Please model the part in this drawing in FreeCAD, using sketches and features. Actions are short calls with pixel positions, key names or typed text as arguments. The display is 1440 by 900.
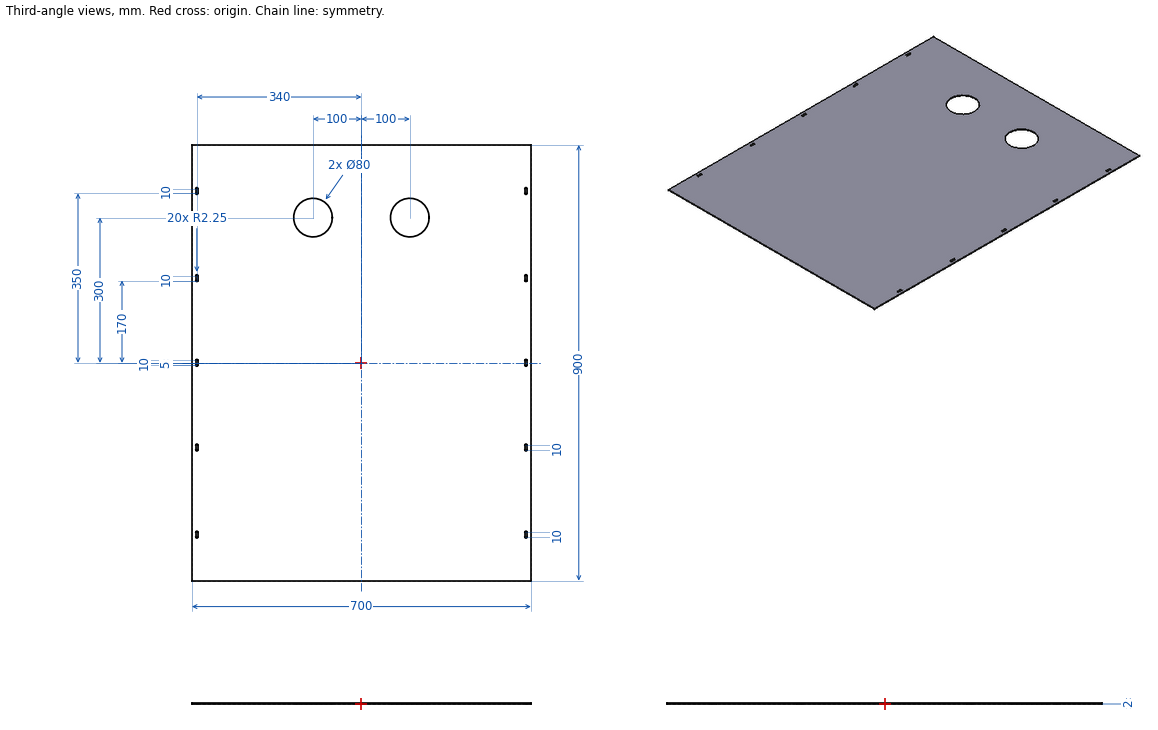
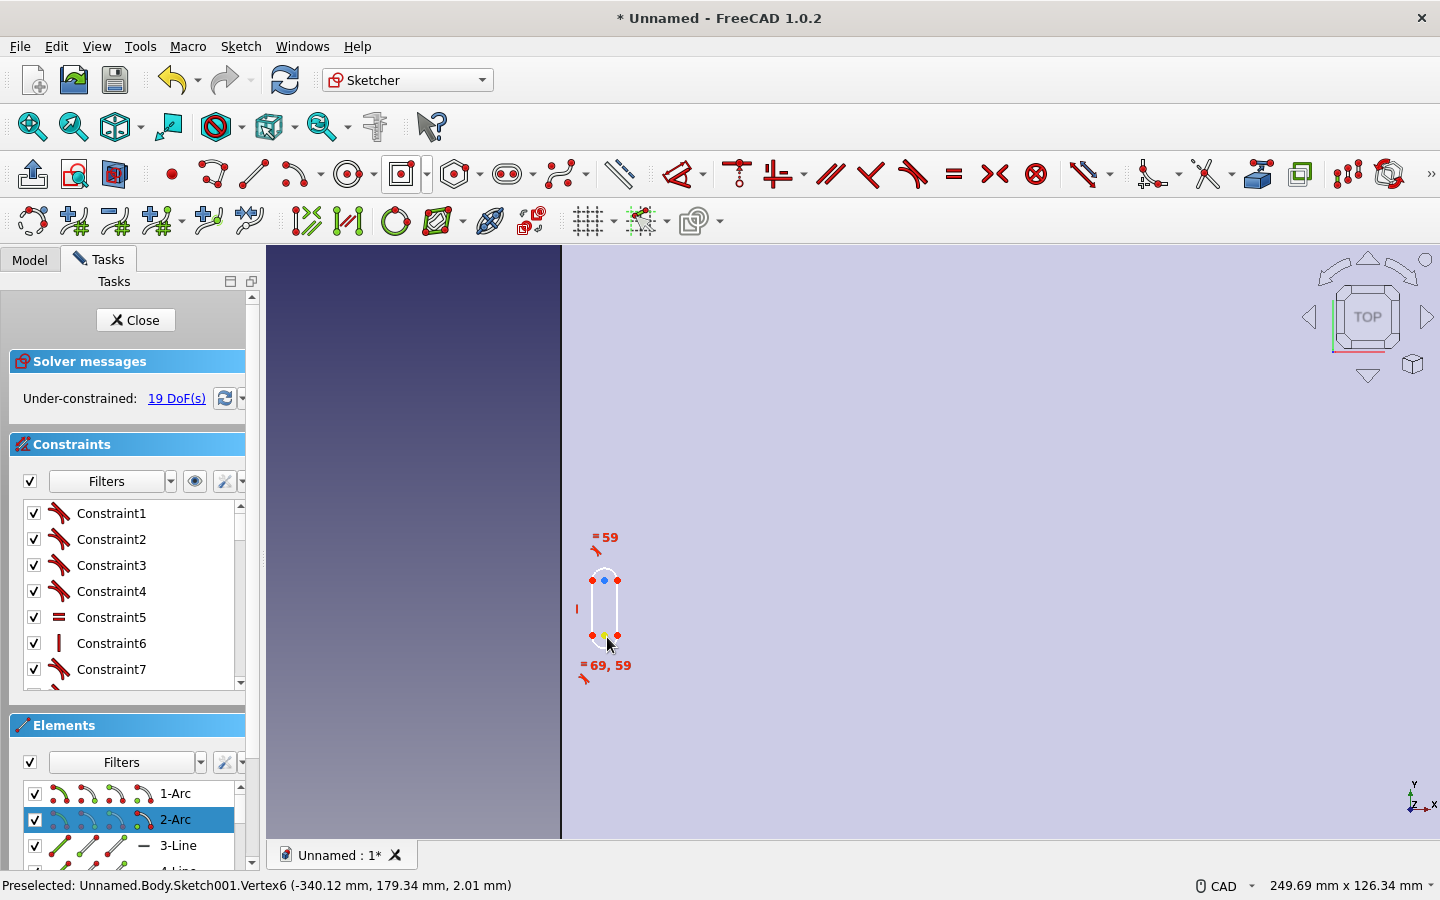
click(605, 636)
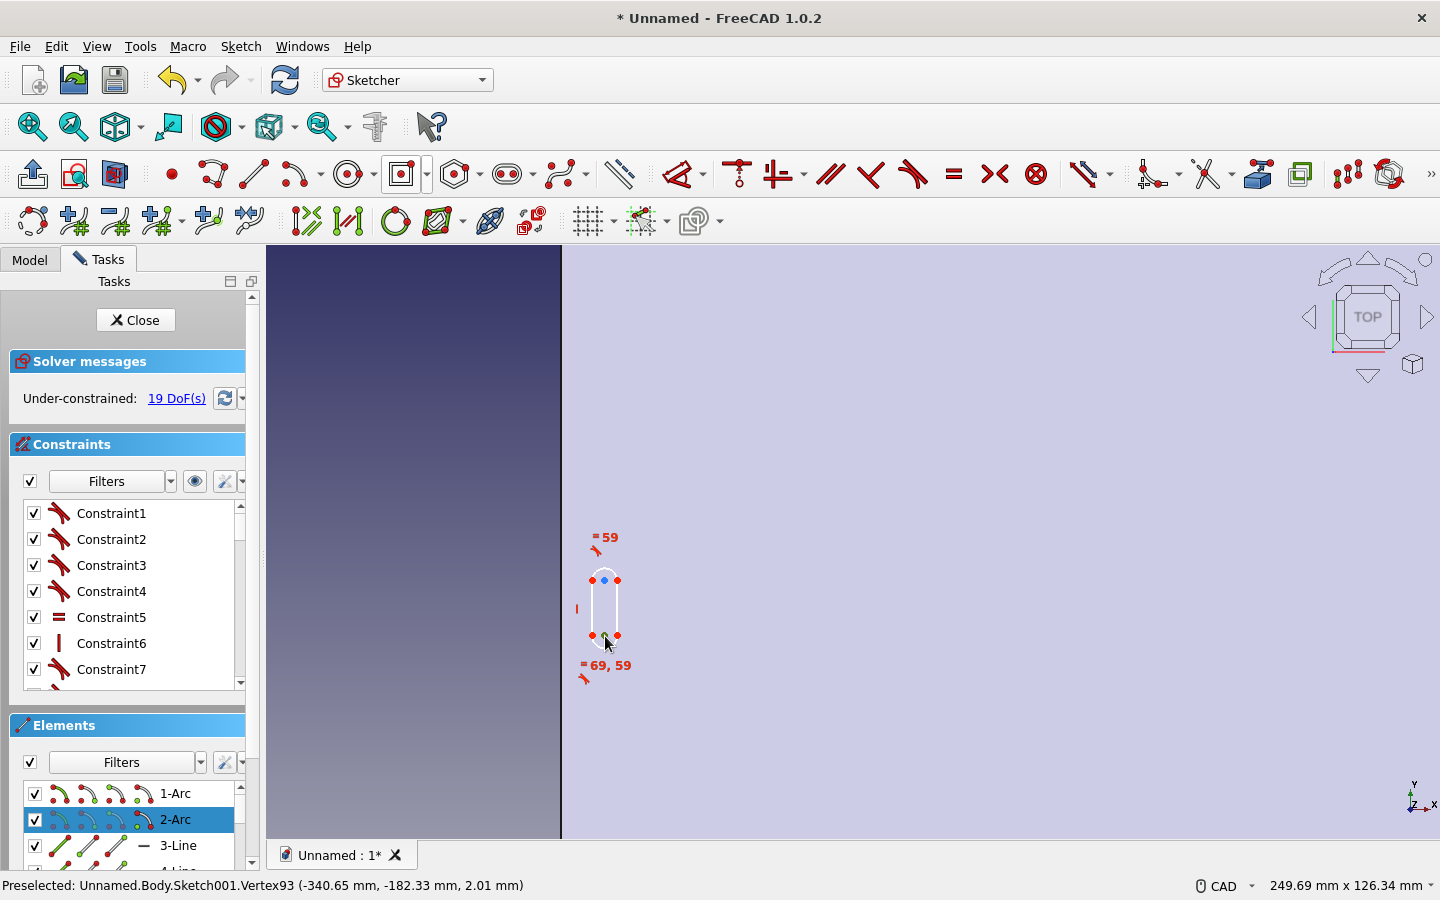
scroll(607, 637, down, 11)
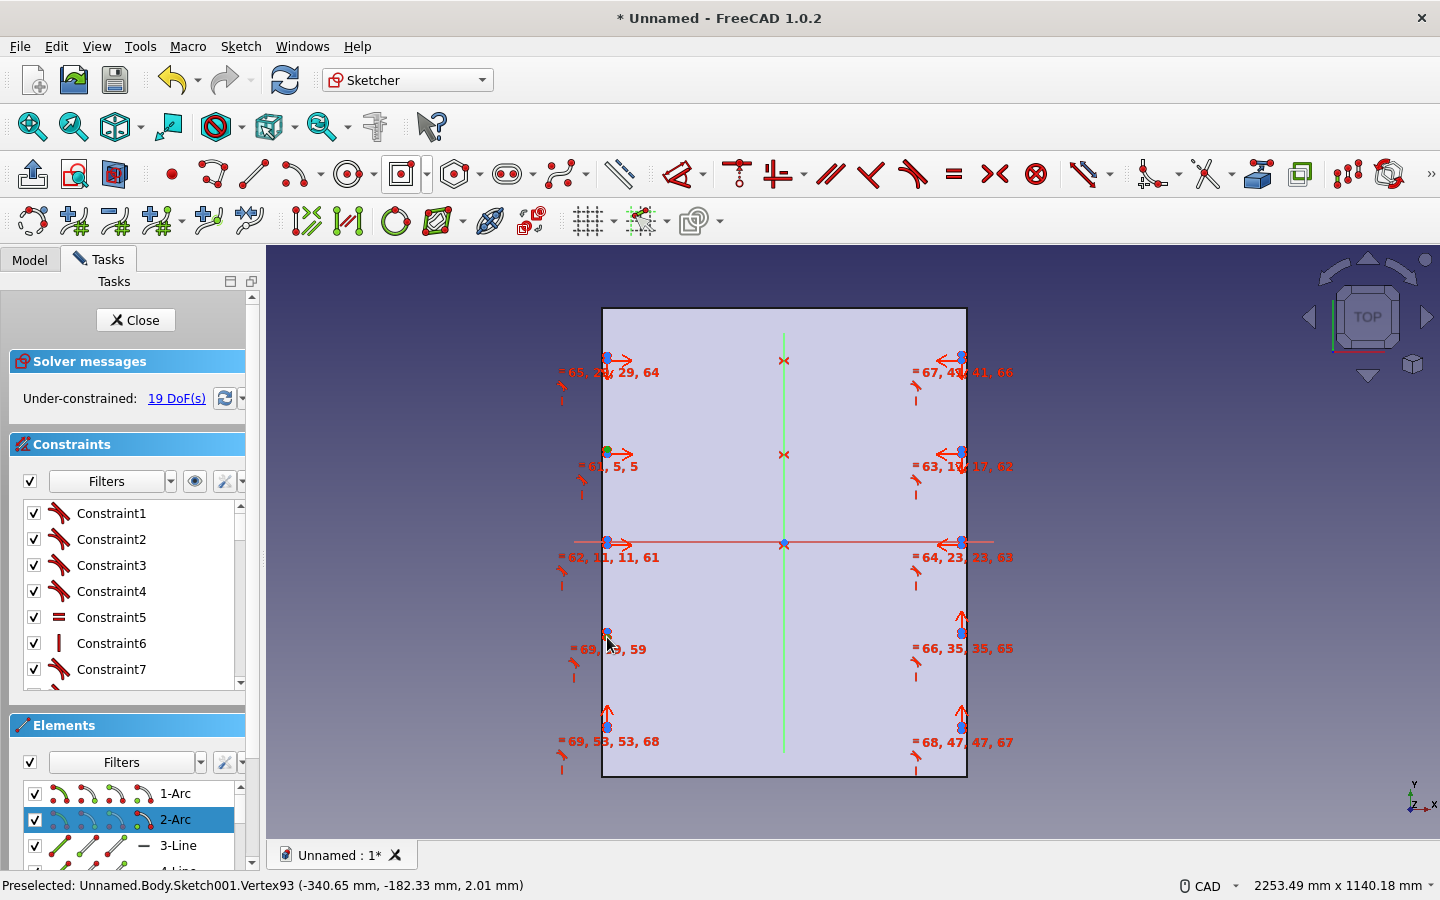
click(574, 542)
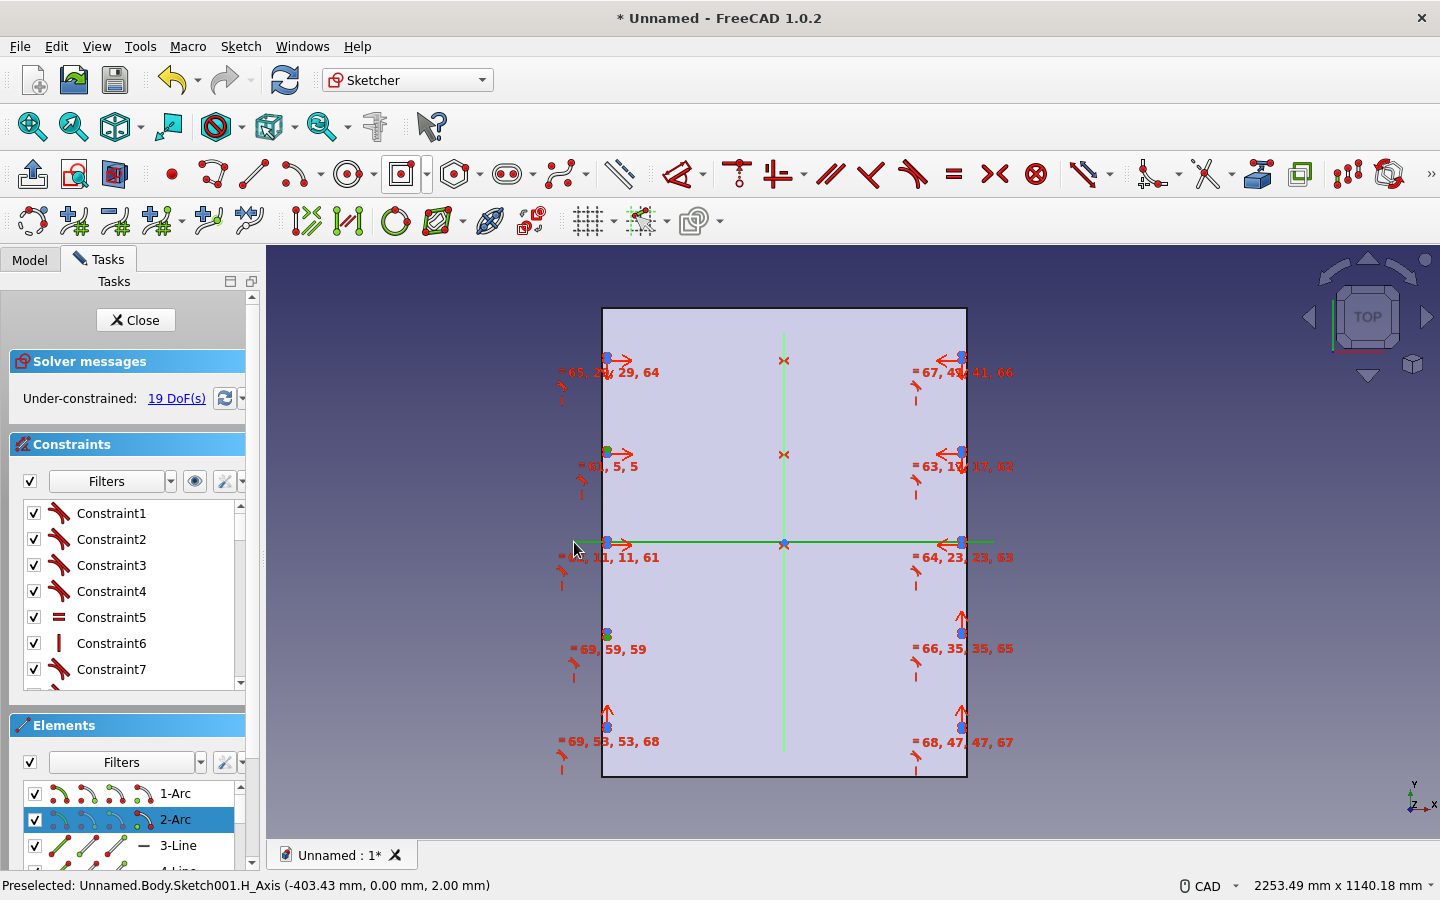
key(s)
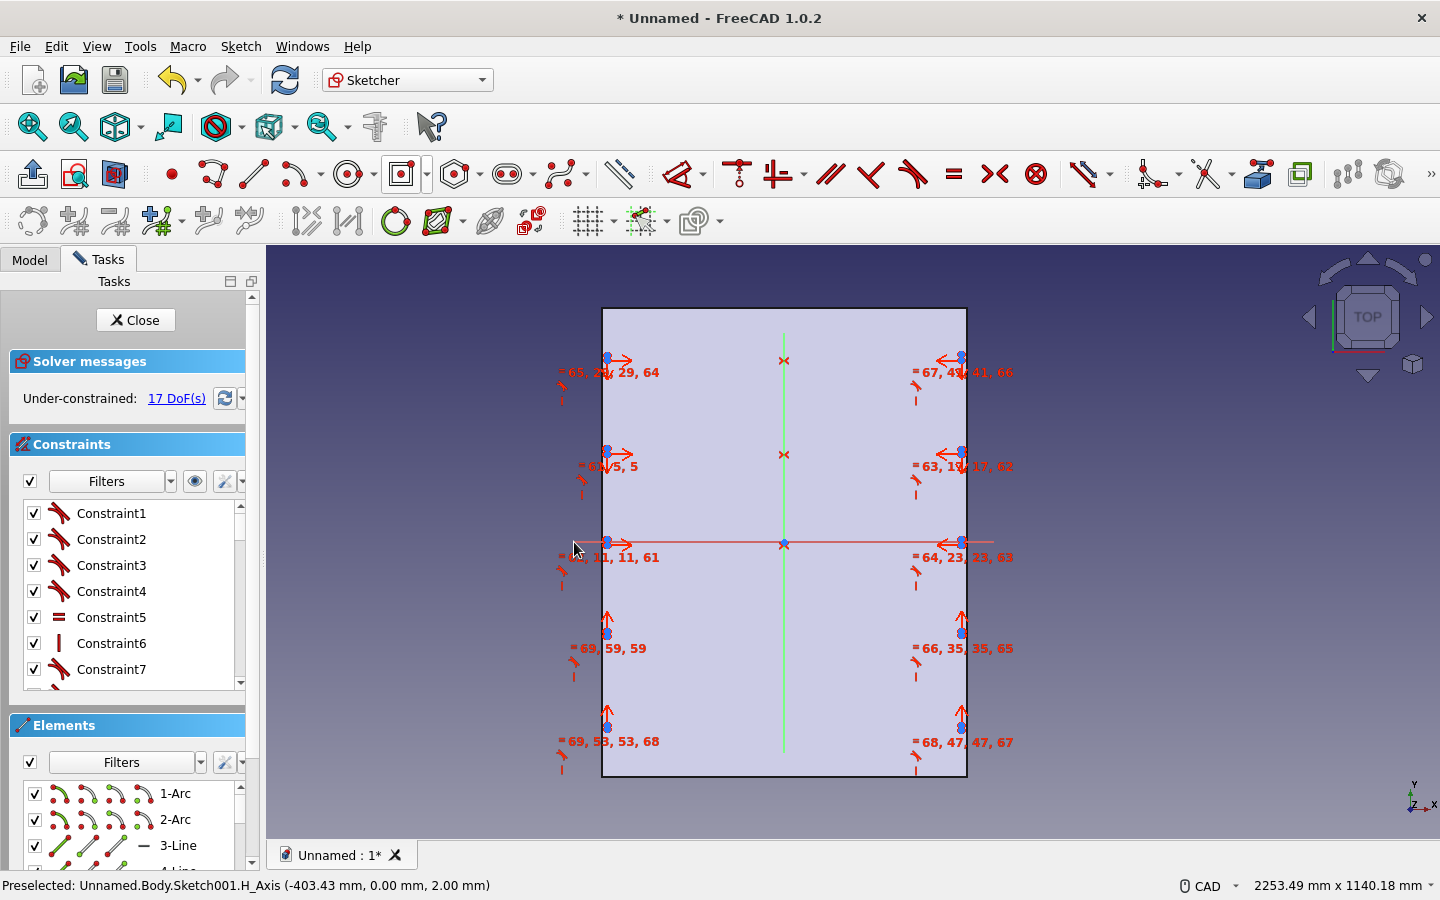
key(d)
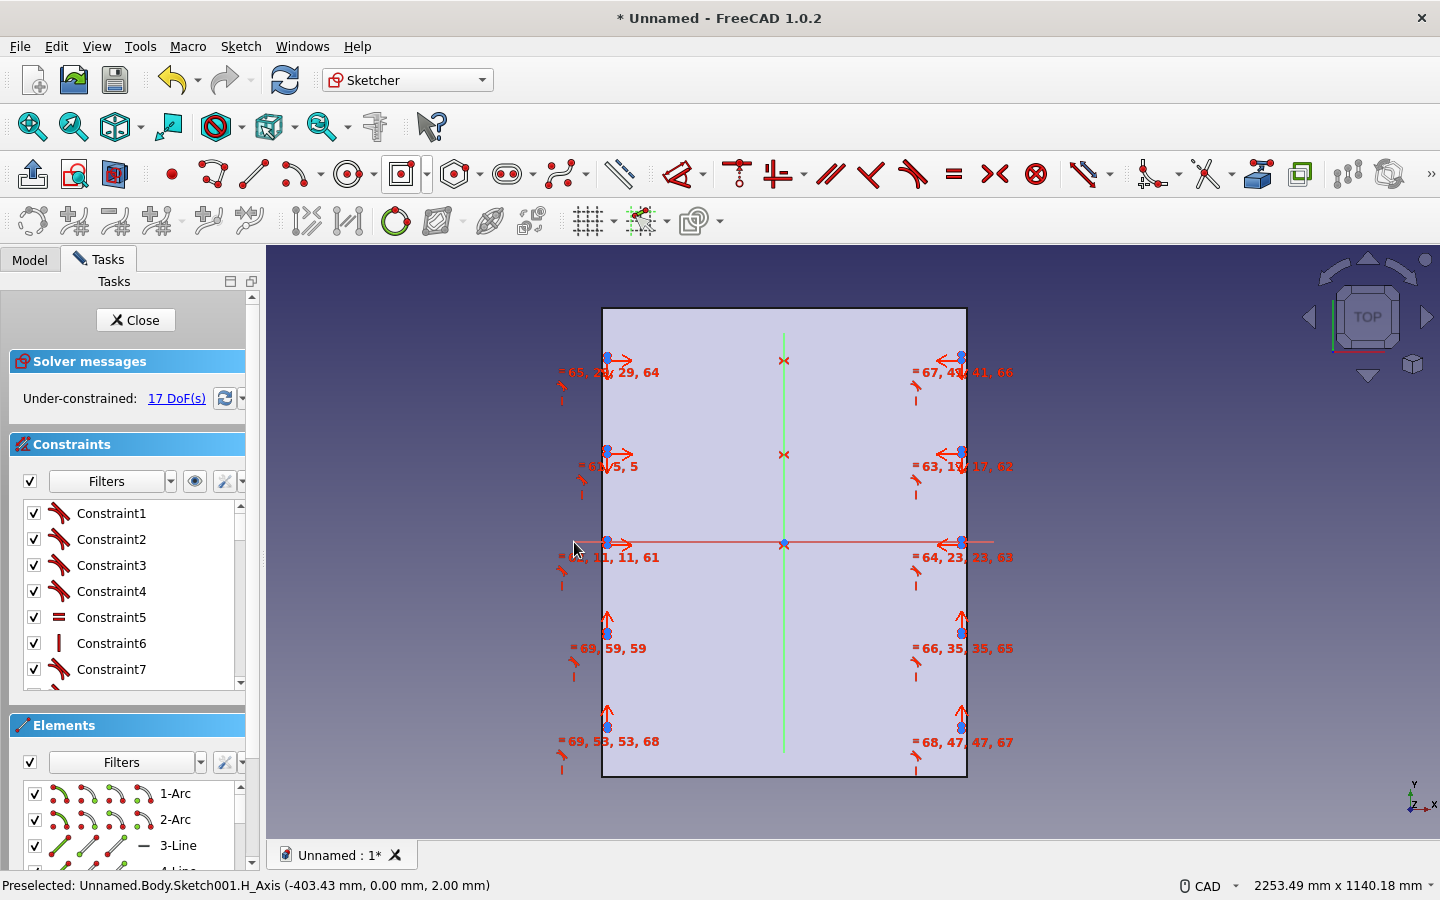
scroll(607, 456, up, 18)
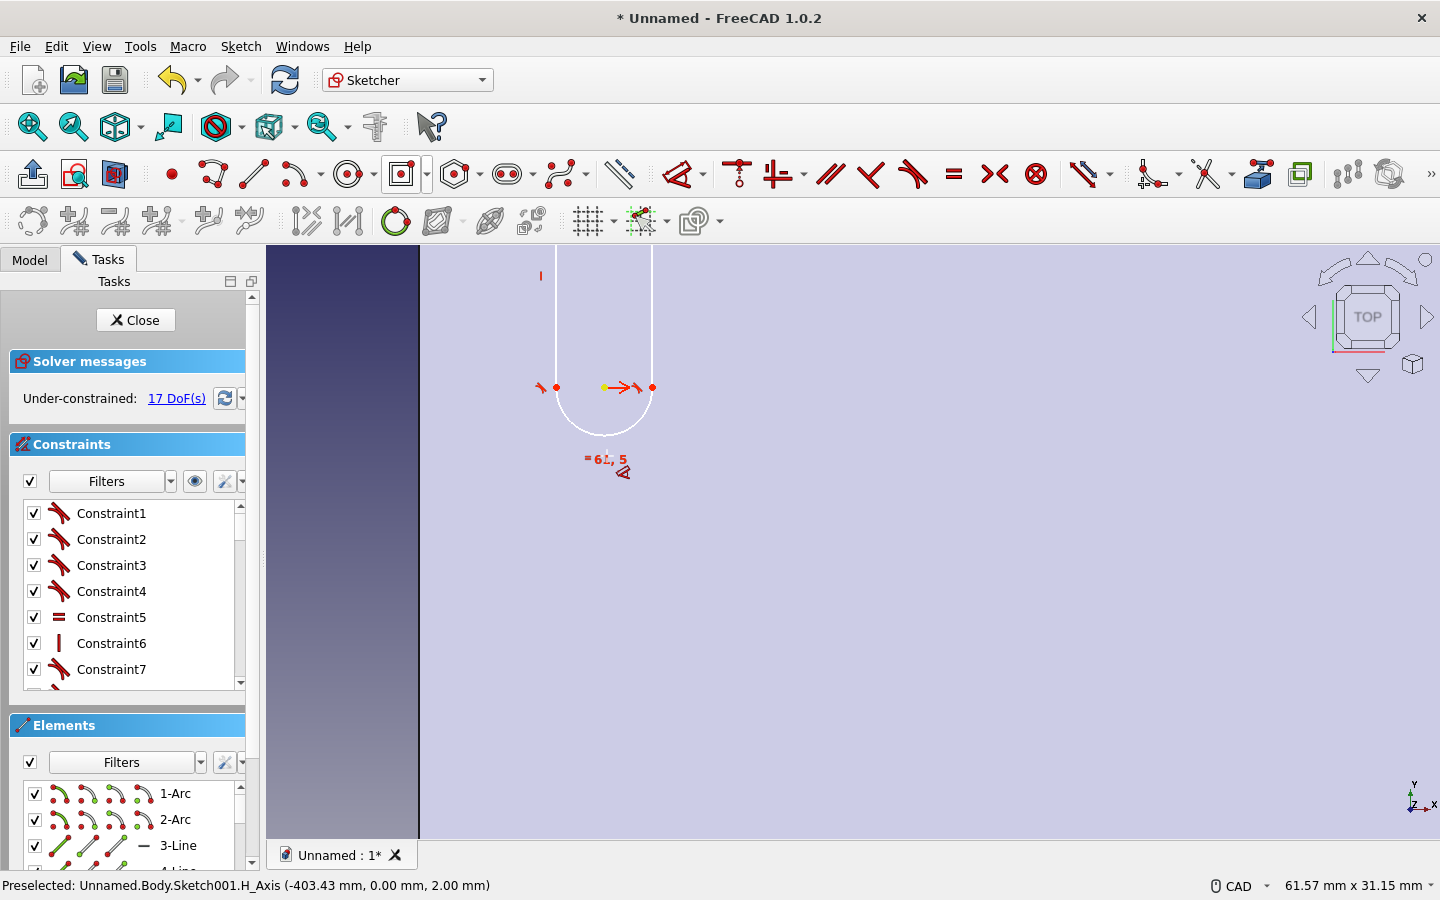
click(604, 436)
click(604, 468)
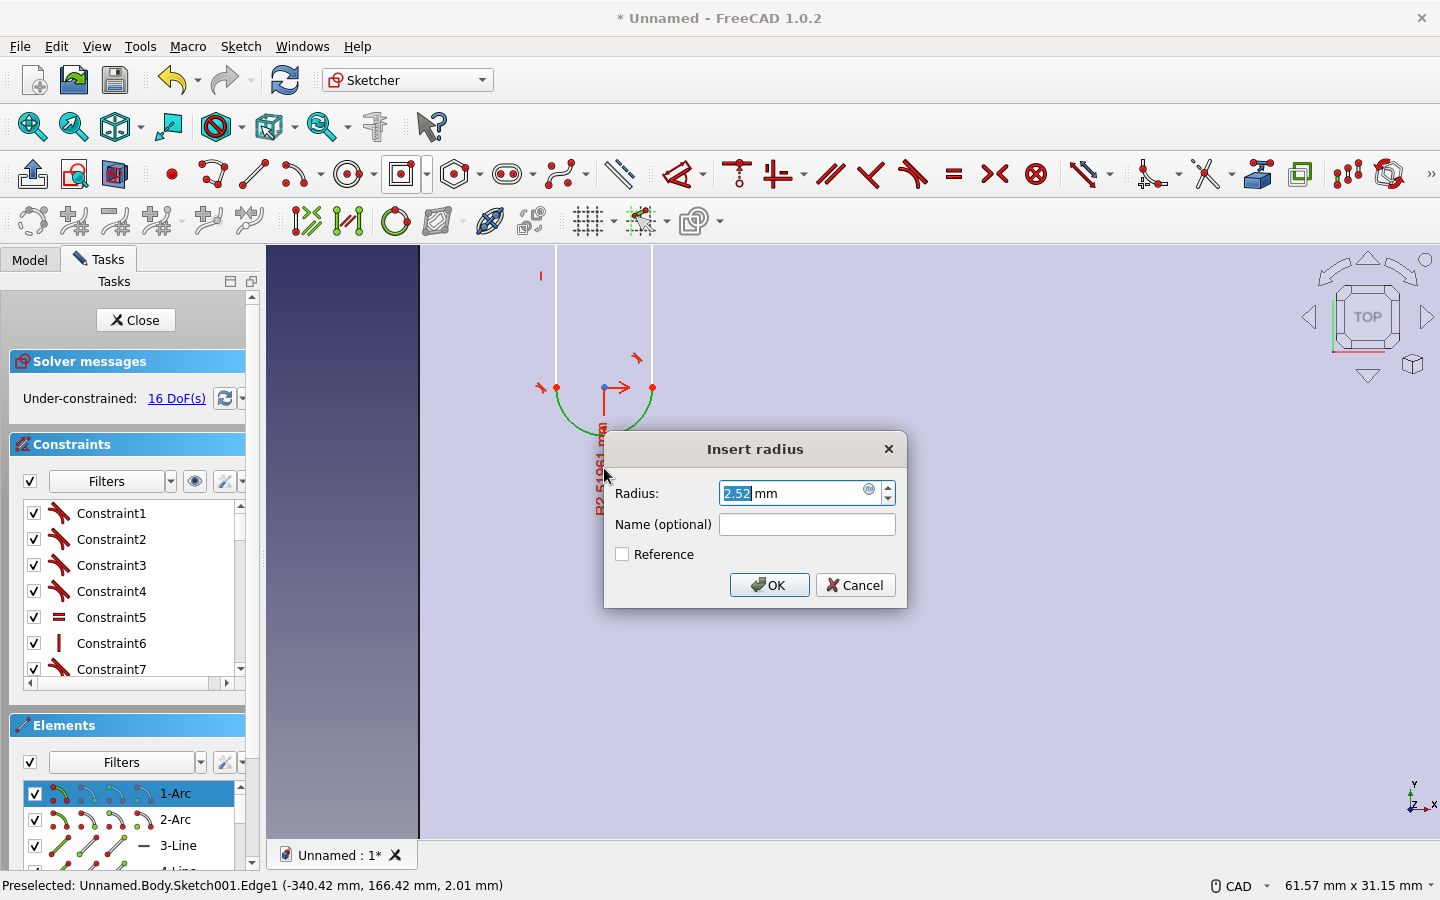
text(2.25)
key(Return)